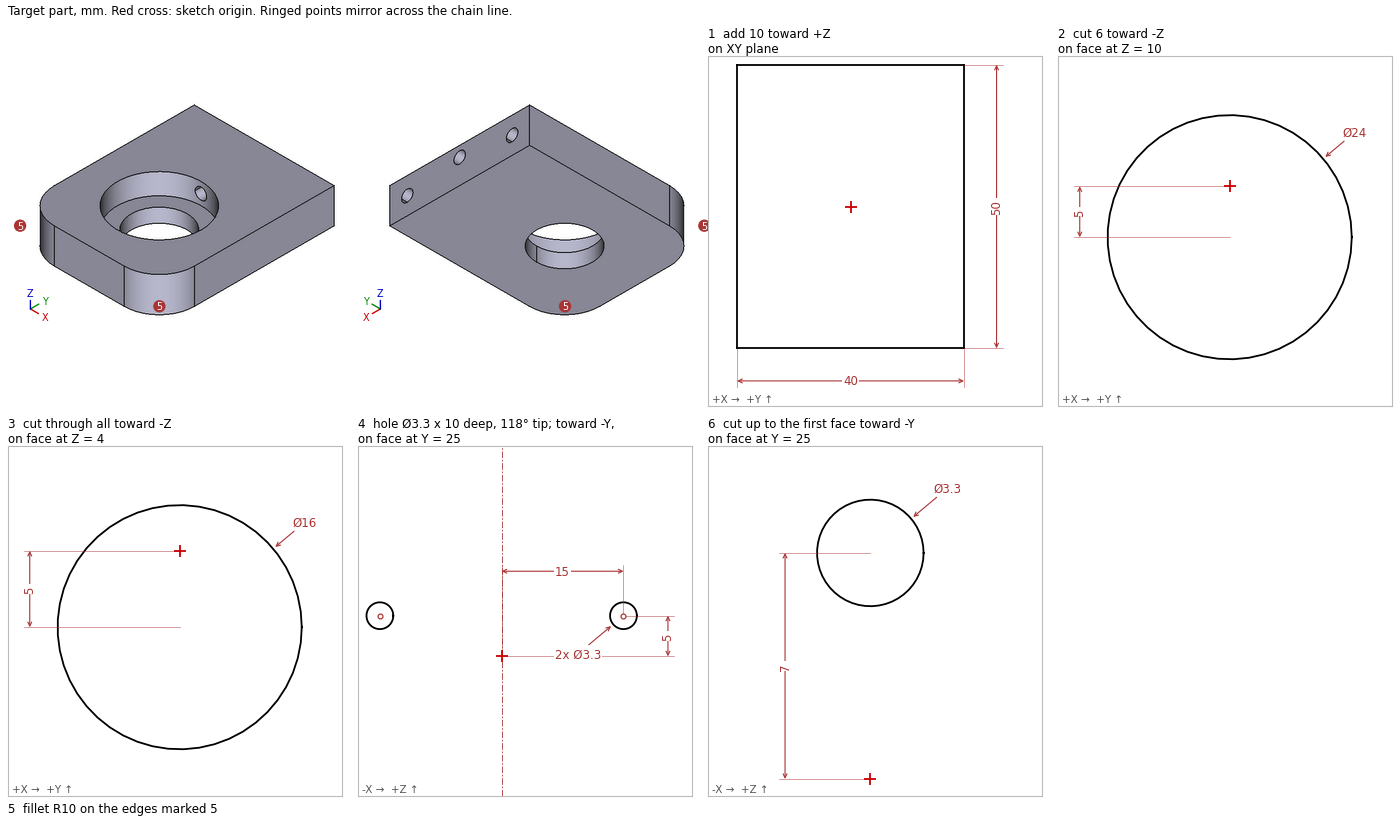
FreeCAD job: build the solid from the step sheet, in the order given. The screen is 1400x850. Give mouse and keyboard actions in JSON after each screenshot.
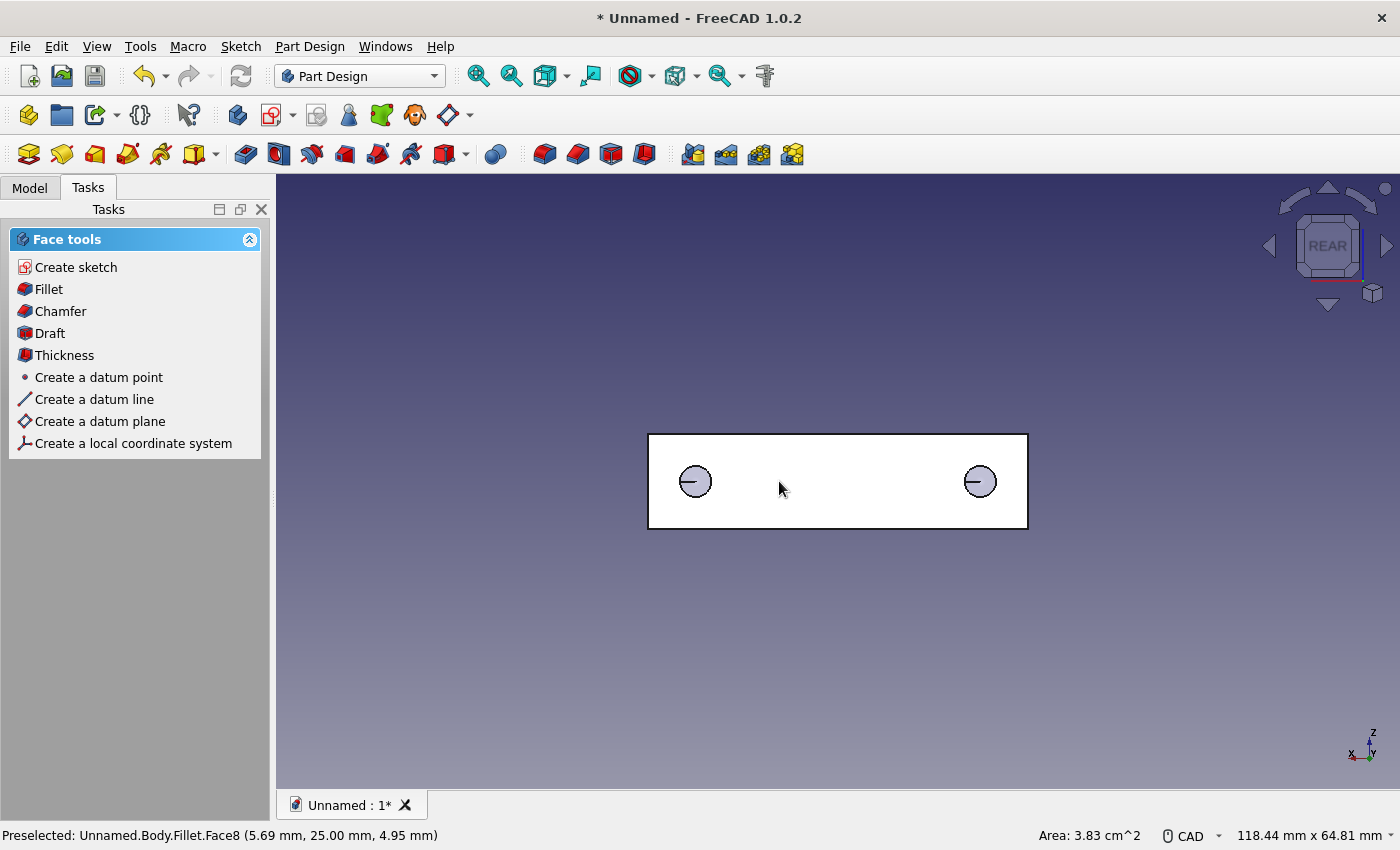
{"action": "left_click", "coordinate": [270, 116]}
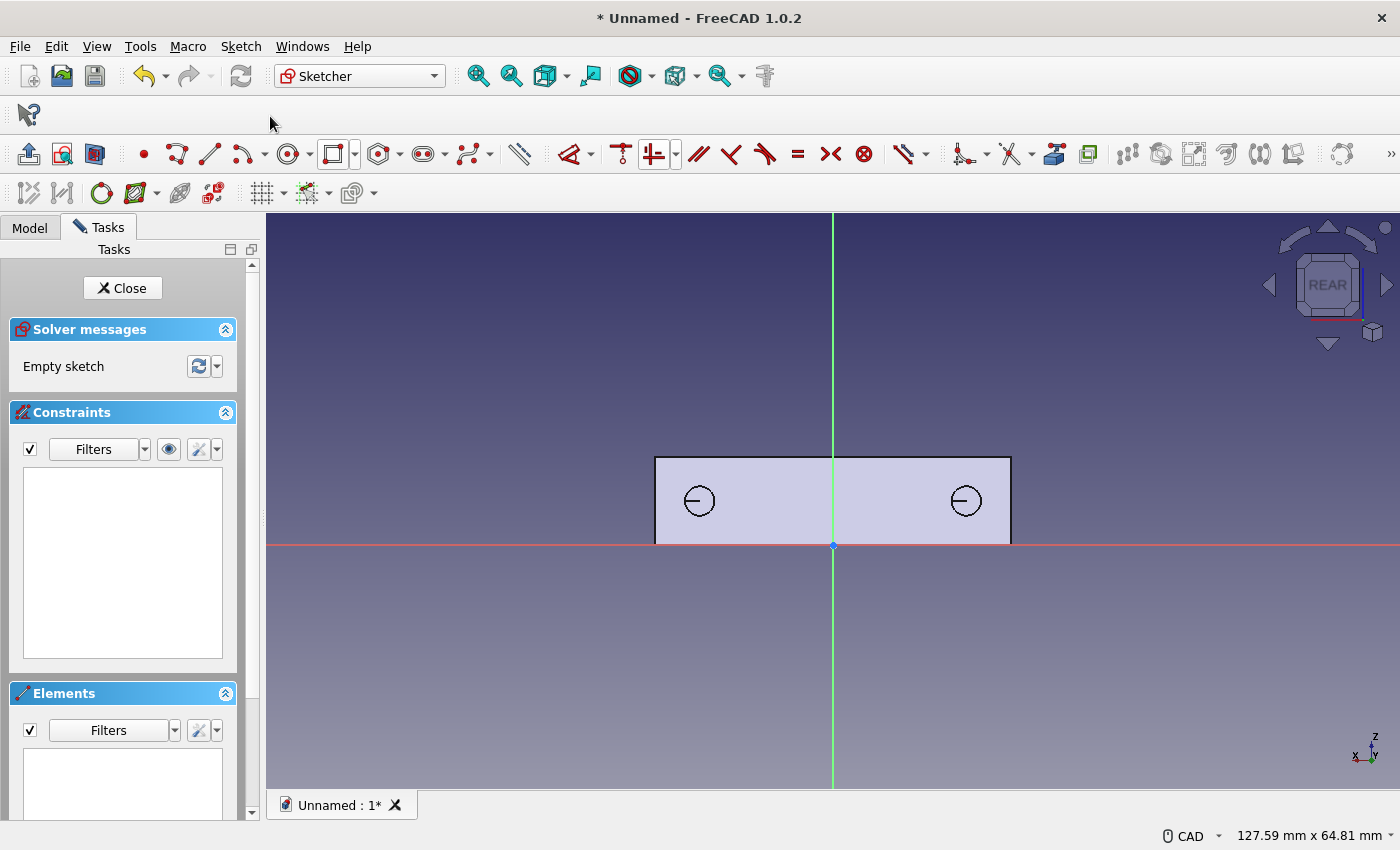
{"action": "scroll", "coordinate": [838, 482], "scroll_direction": "up", "scroll_amount": 13}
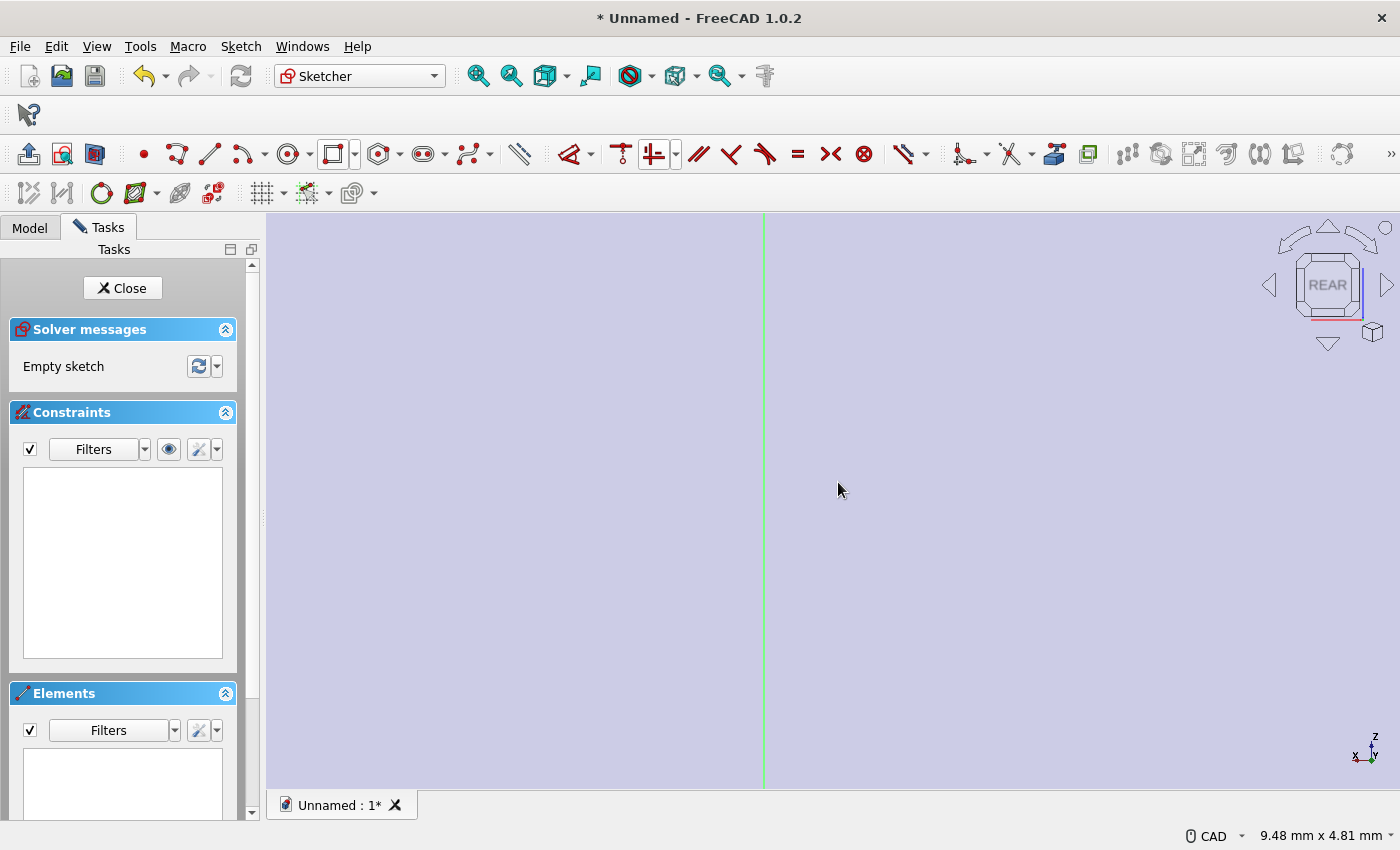
{"action": "left_click", "coordinate": [288, 154]}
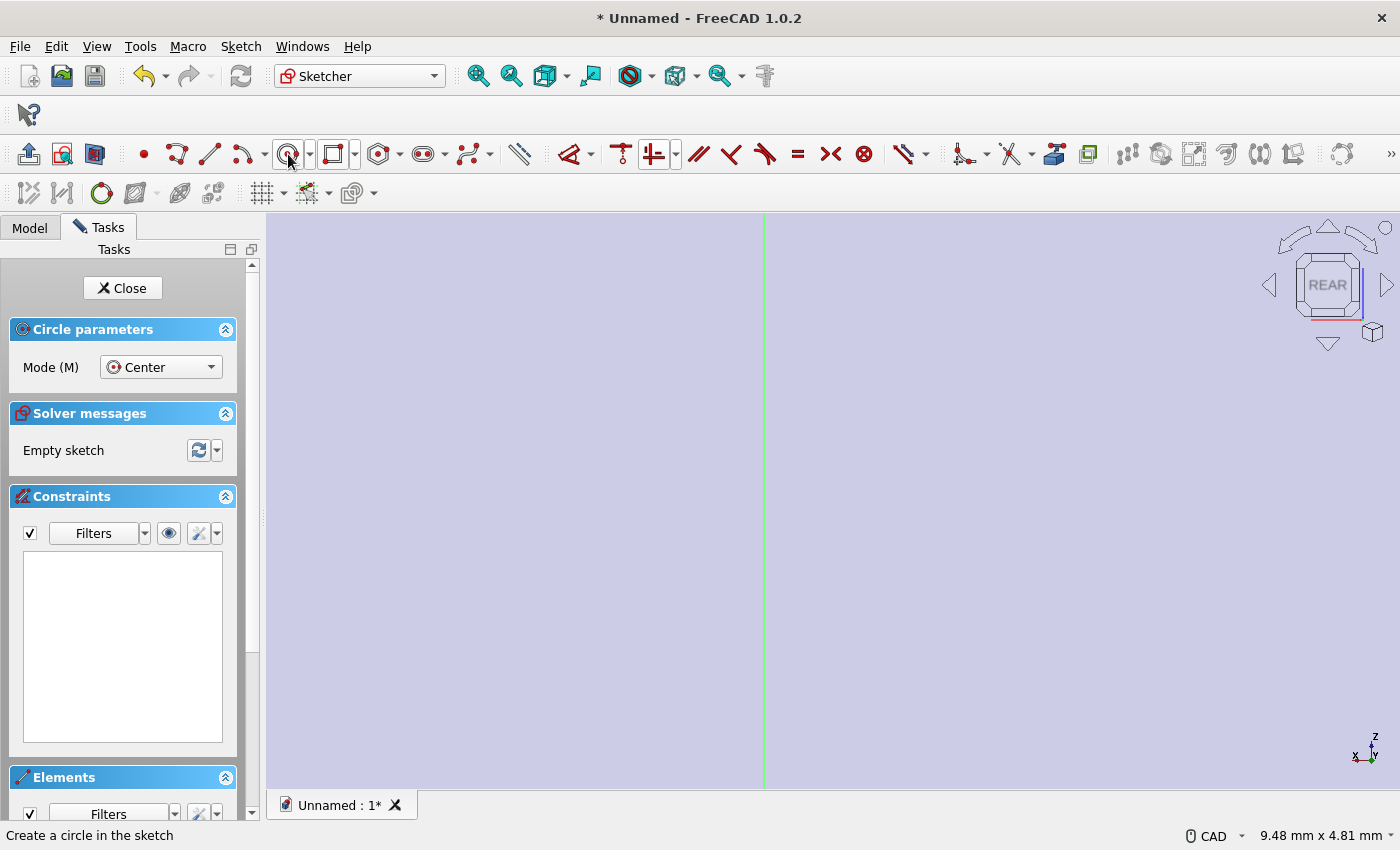
{"action": "left_click", "coordinate": [764, 493]}
{"action": "mouse_move", "coordinate": [904, 353]}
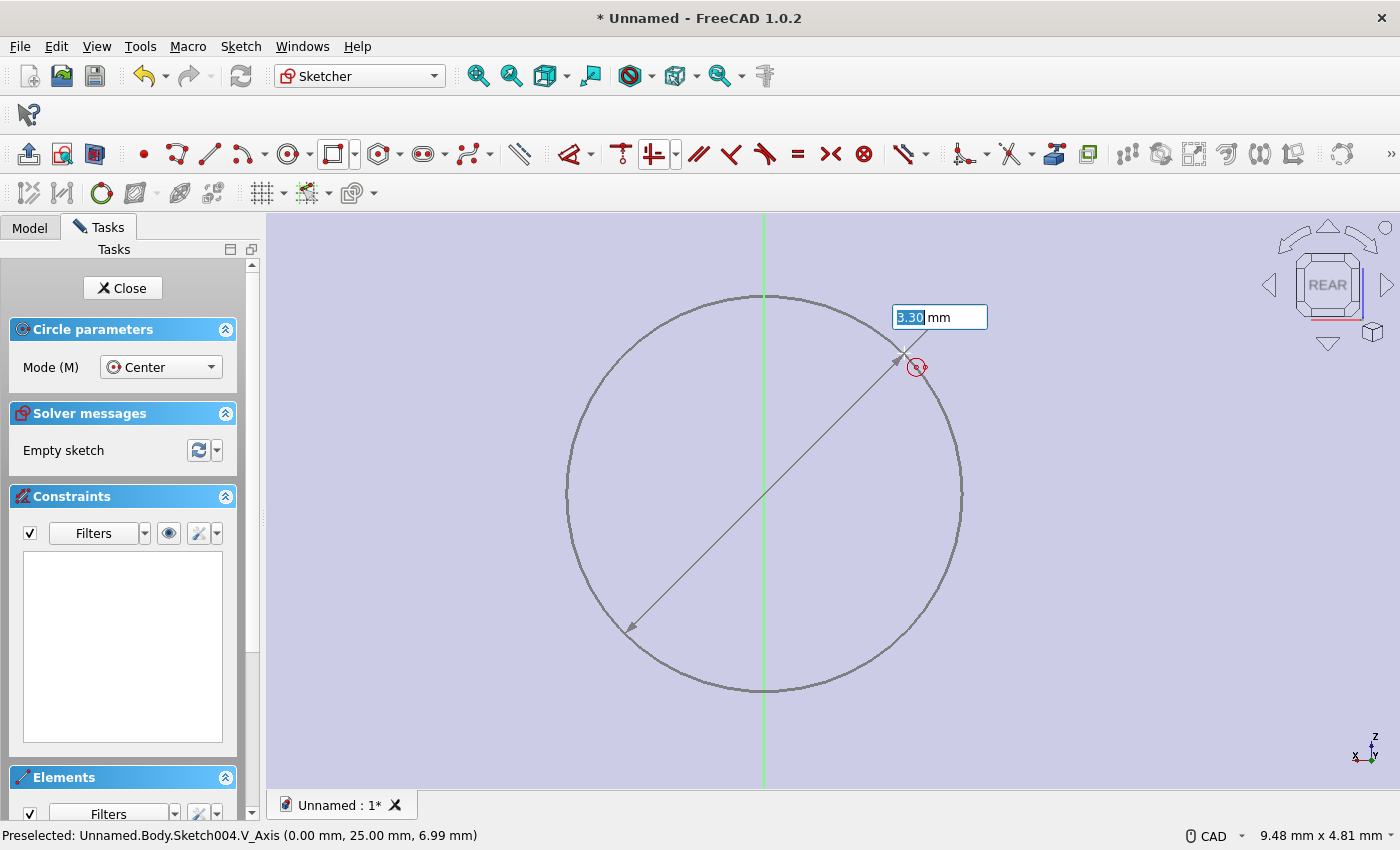
{"action": "type", "text": "3.3"}
{"action": "key", "text": "Return"}
{"action": "key", "text": "Escape"}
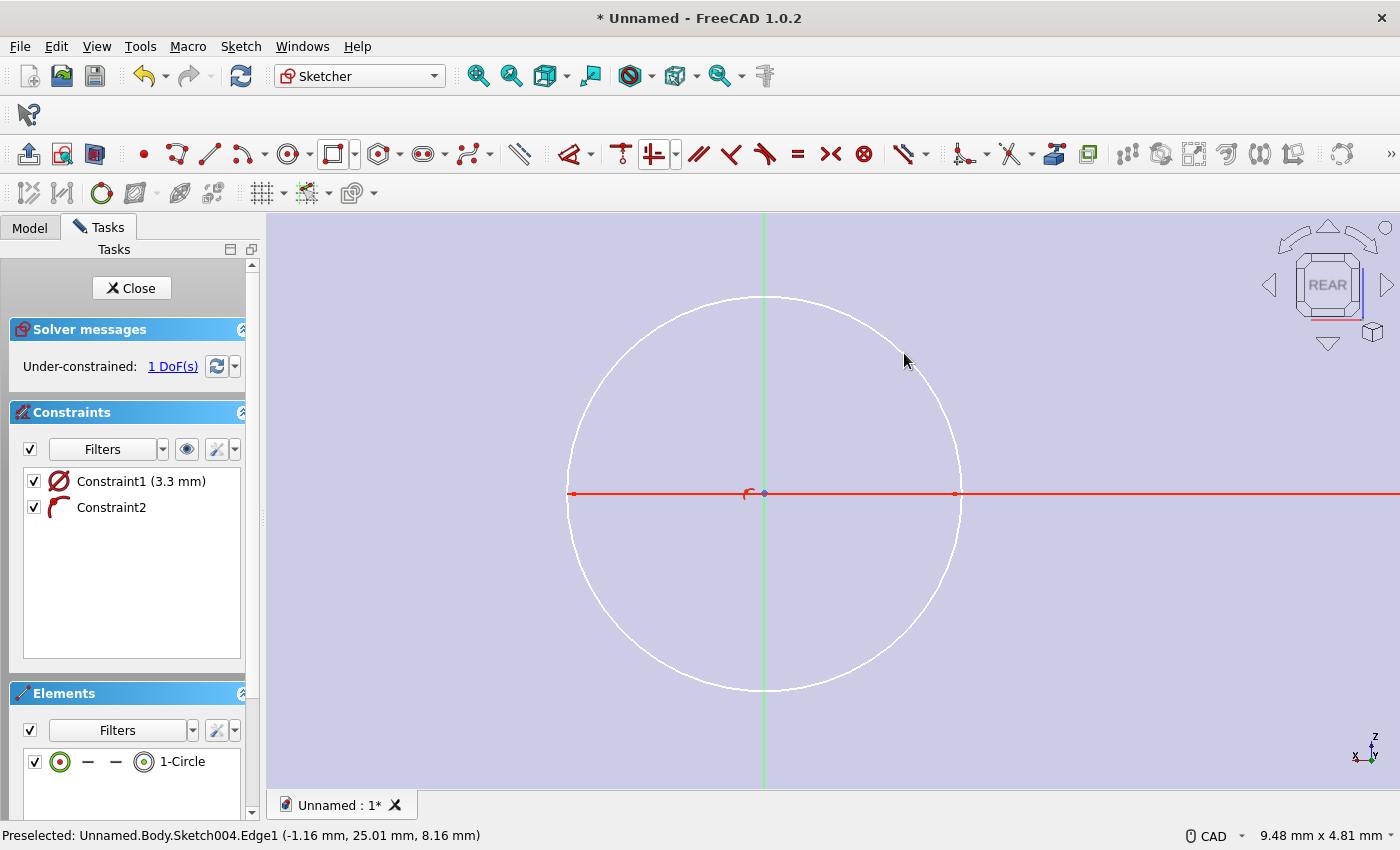
{"action": "left_click", "coordinate": [568, 154]}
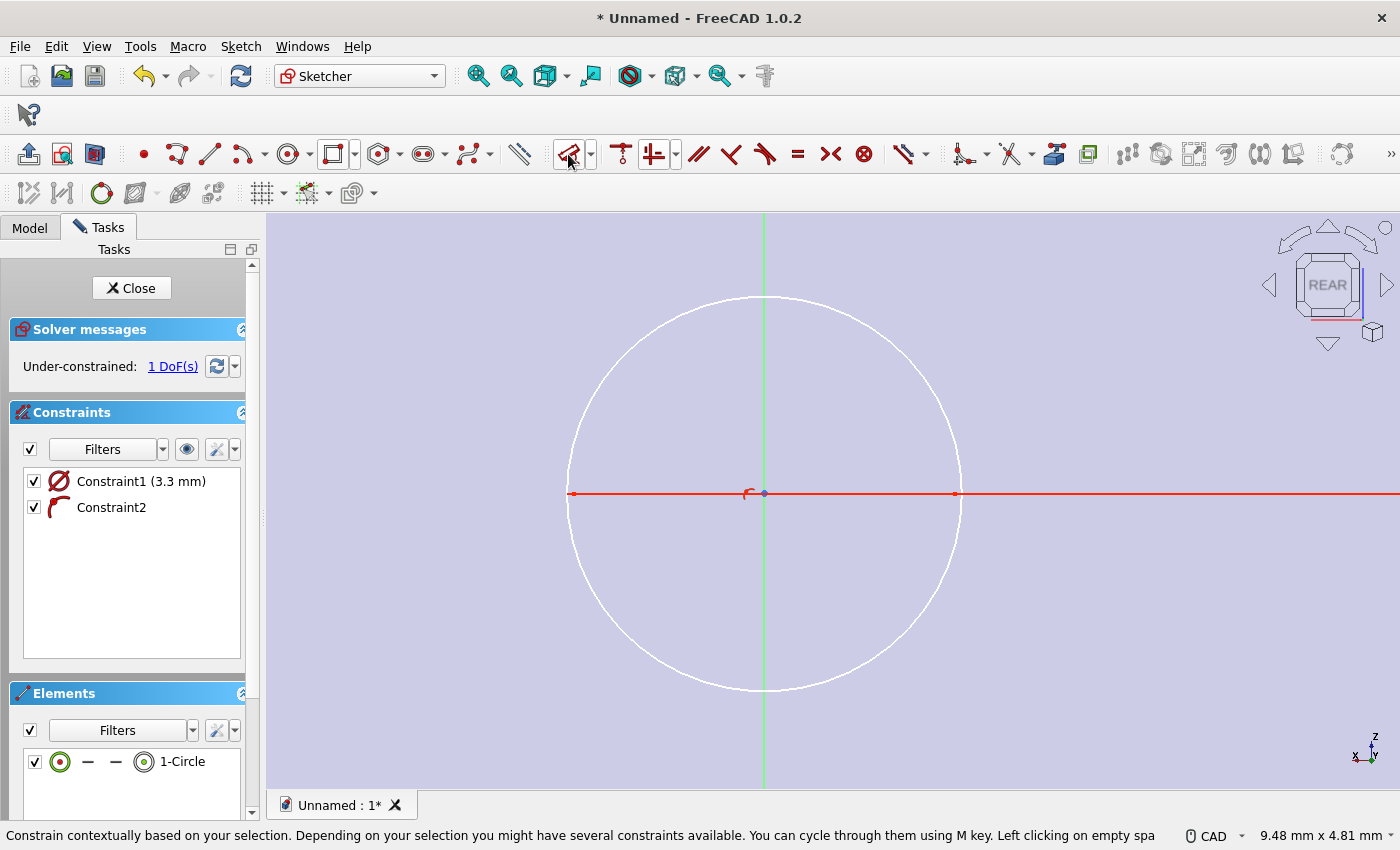
{"action": "left_click", "coordinate": [764, 494]}
{"action": "left_click", "coordinate": [798, 627]}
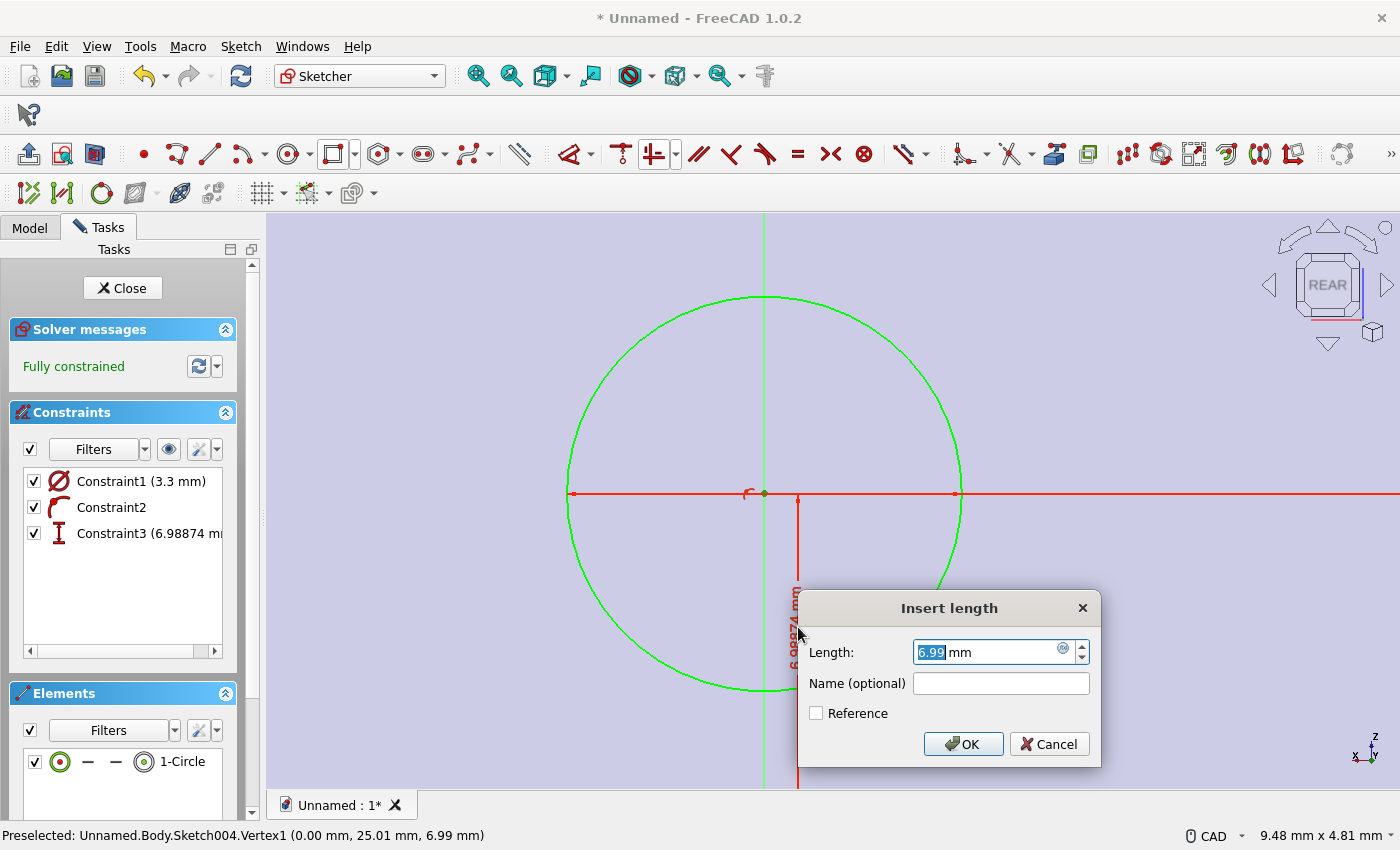
{"action": "type", "text": "7"}
{"action": "key", "text": "Return"}
{"action": "key", "text": "Escape"}